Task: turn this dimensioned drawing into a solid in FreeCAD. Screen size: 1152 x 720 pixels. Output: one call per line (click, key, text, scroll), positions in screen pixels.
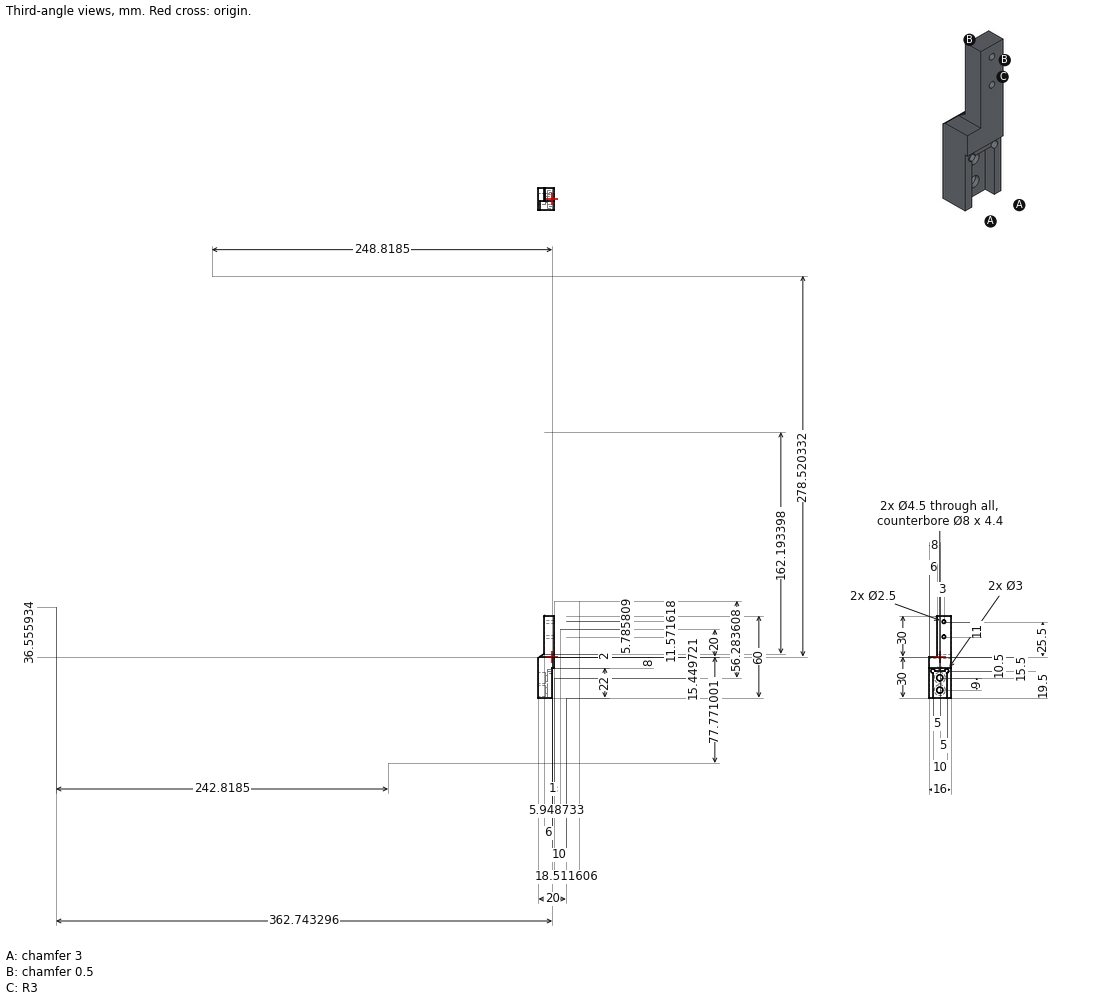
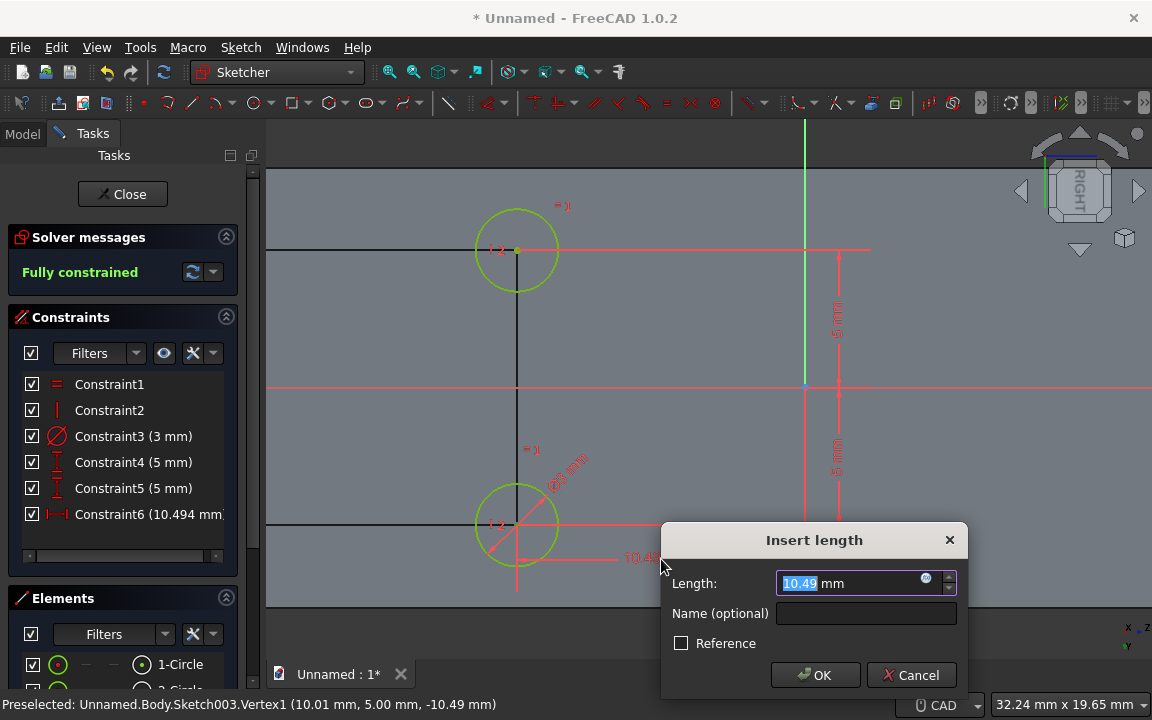
text(10.5)
key(Return)
key(Escape)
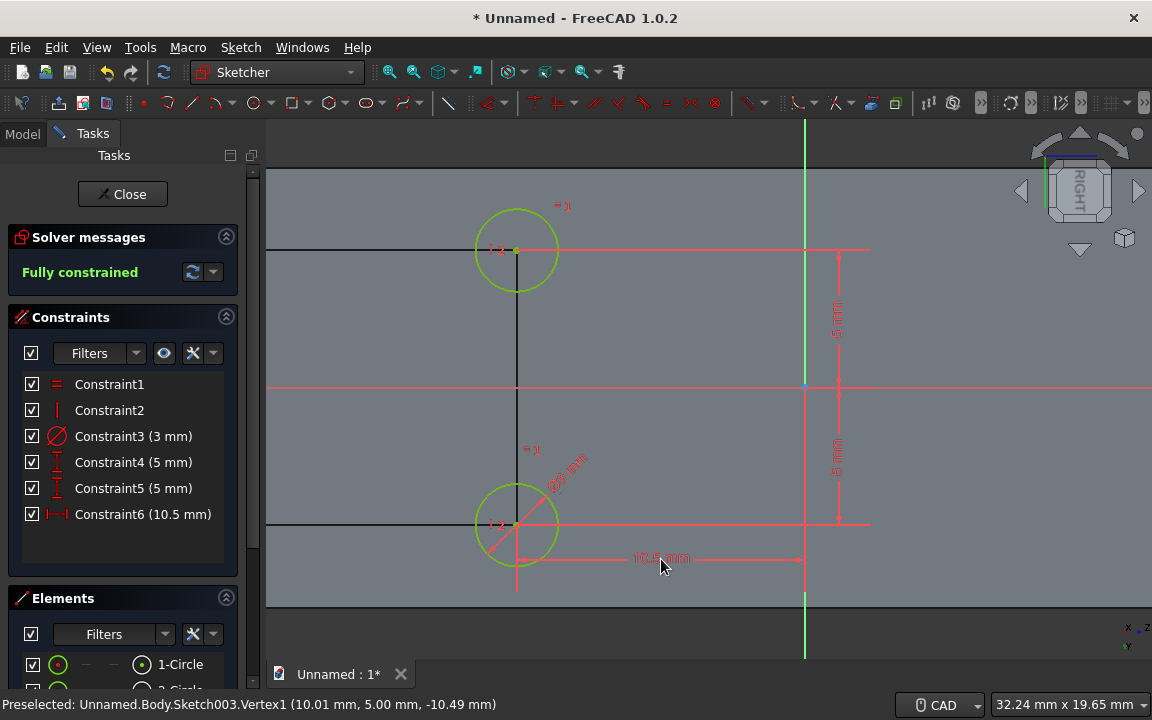
click(123, 194)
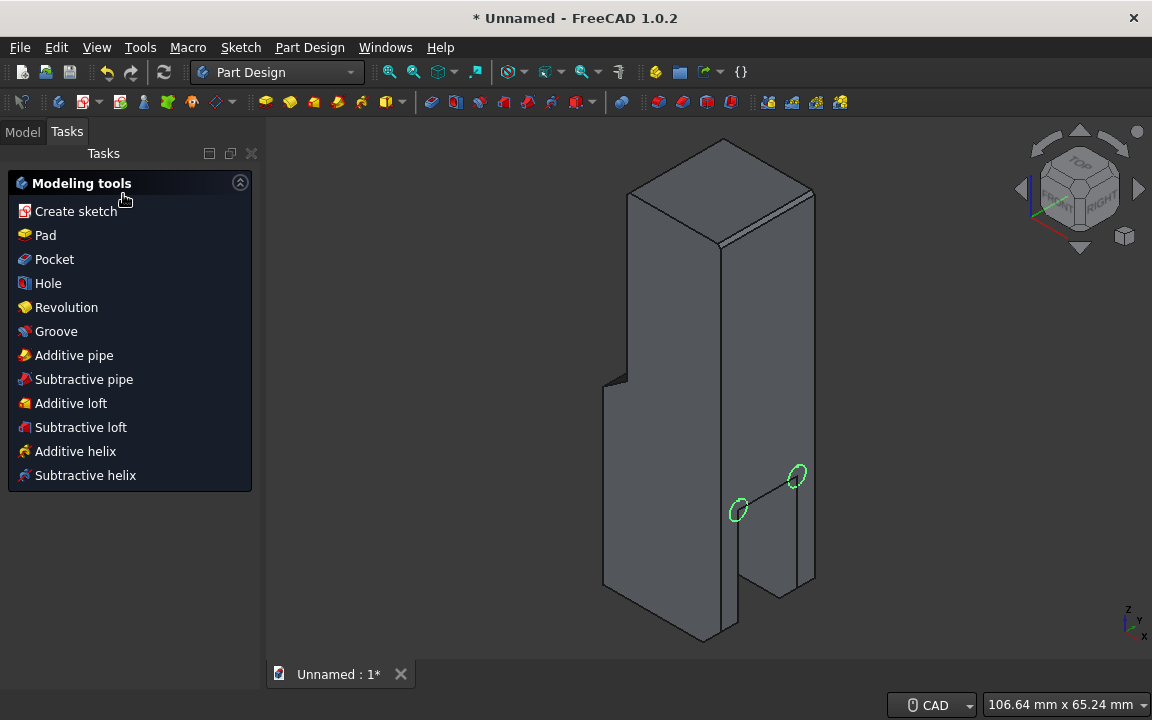
click(432, 102)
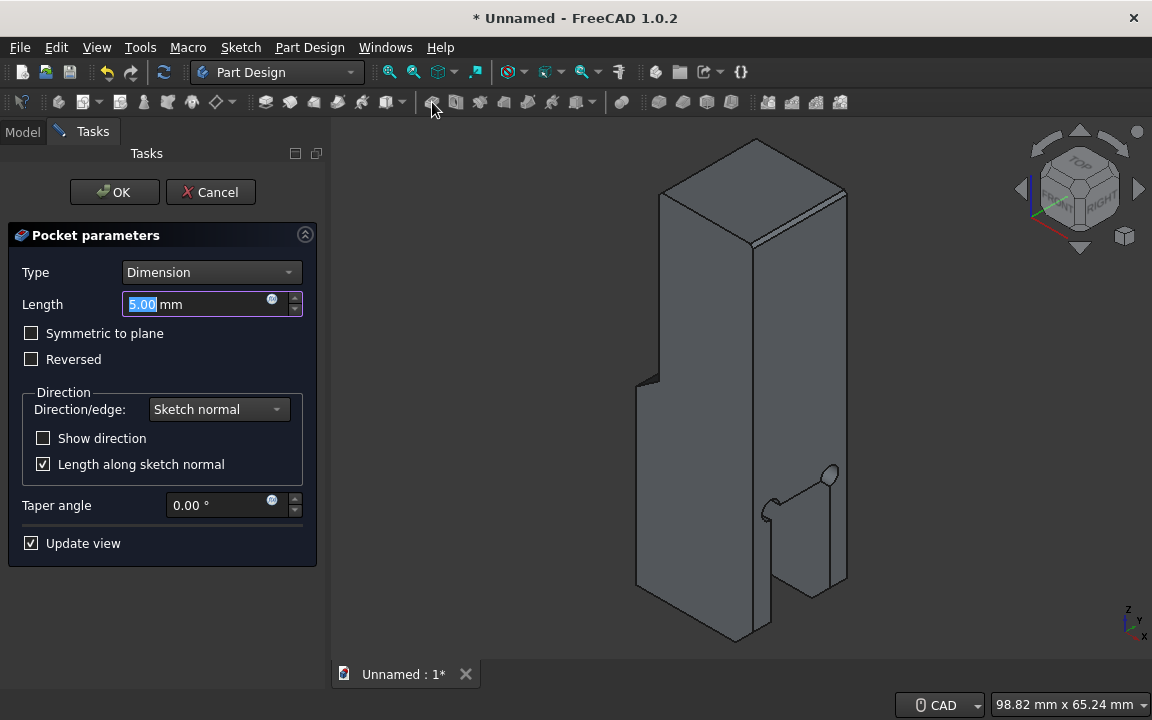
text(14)
key(Tab)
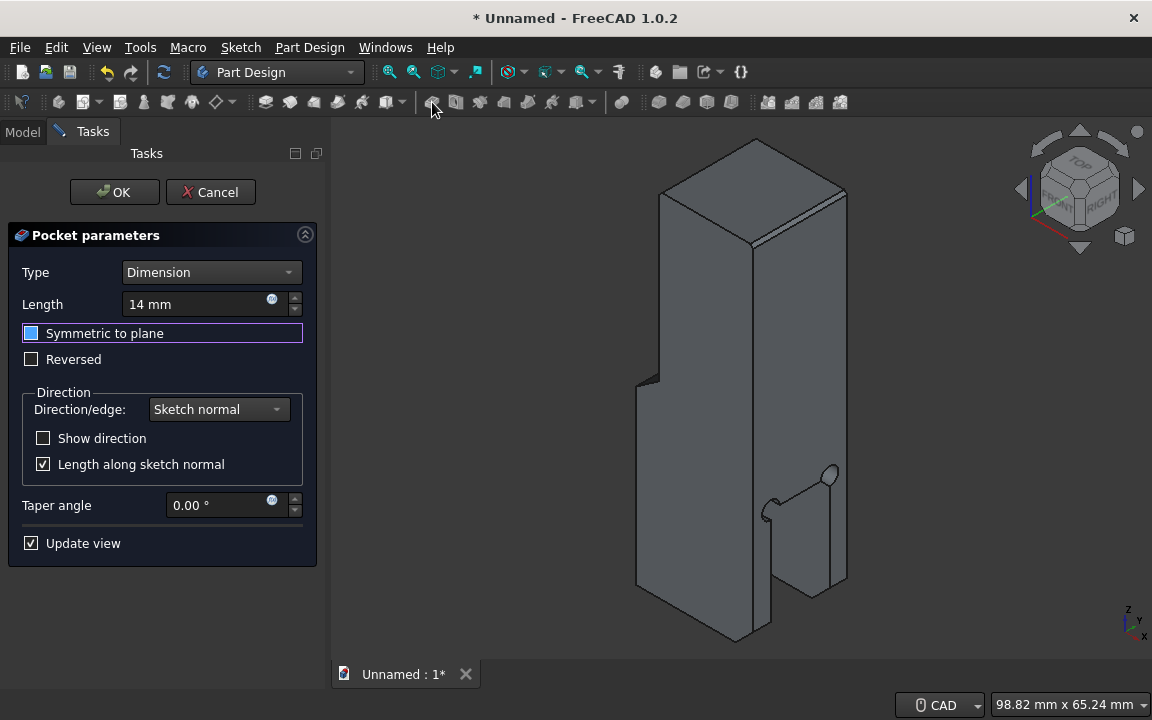
click(115, 192)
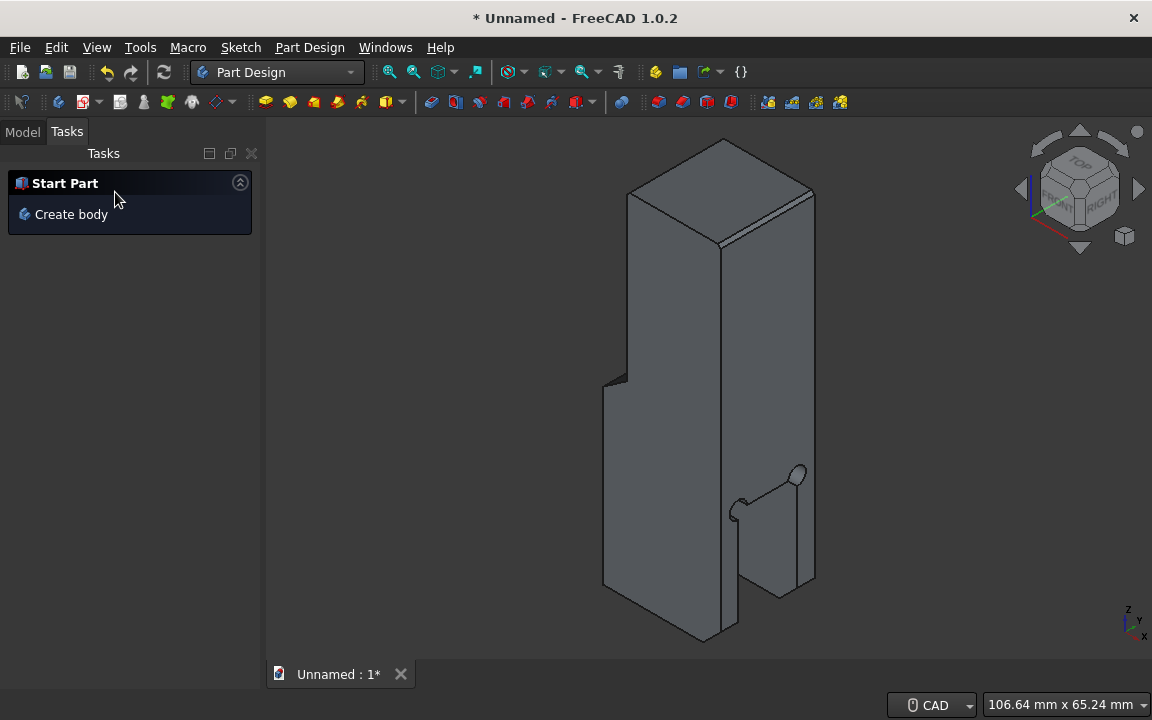
key(6)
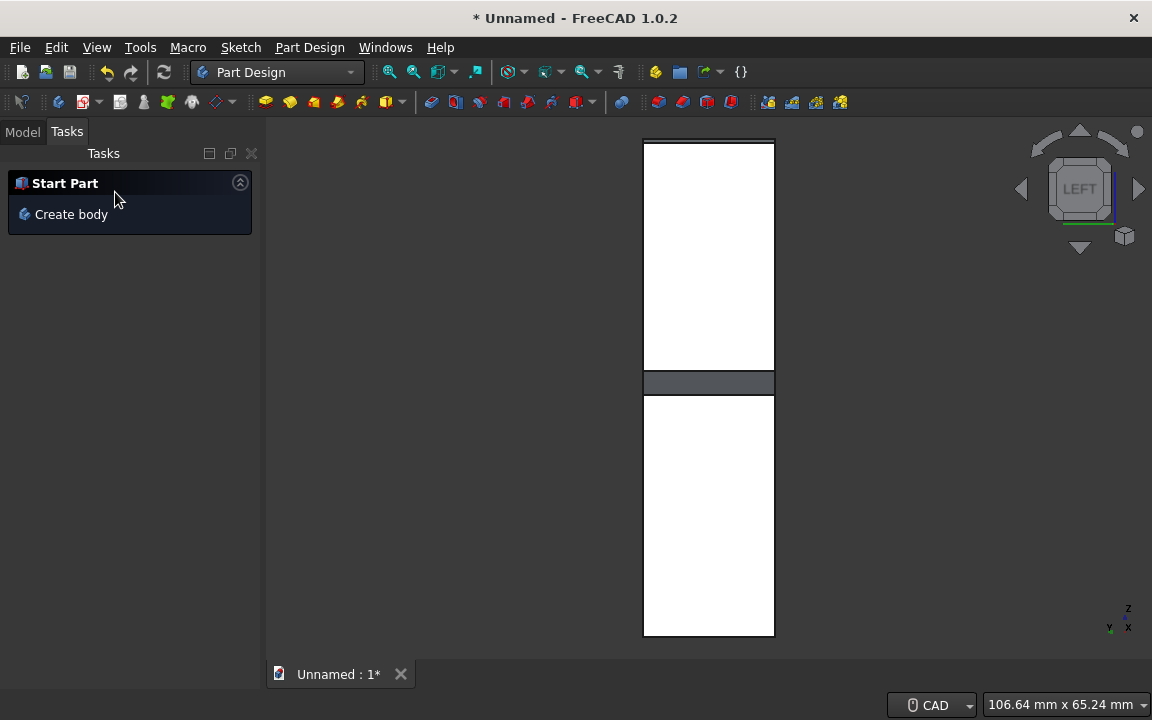
click(709, 480)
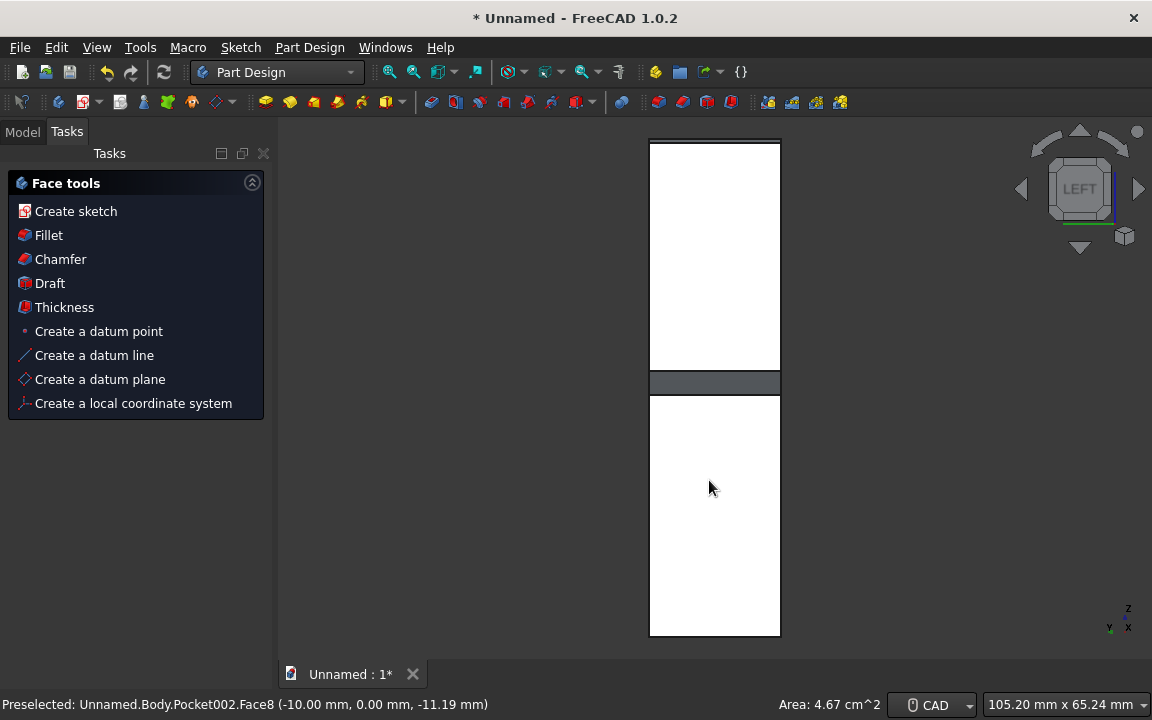
click(84, 102)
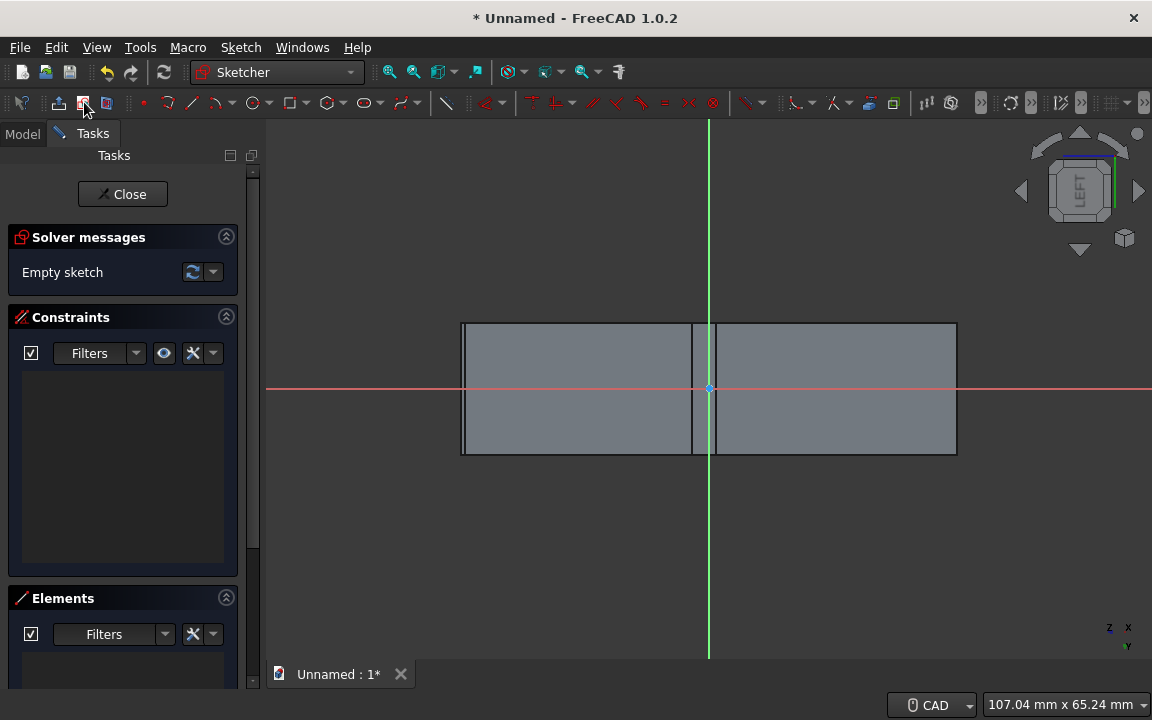
scroll(966, 389, up, 4)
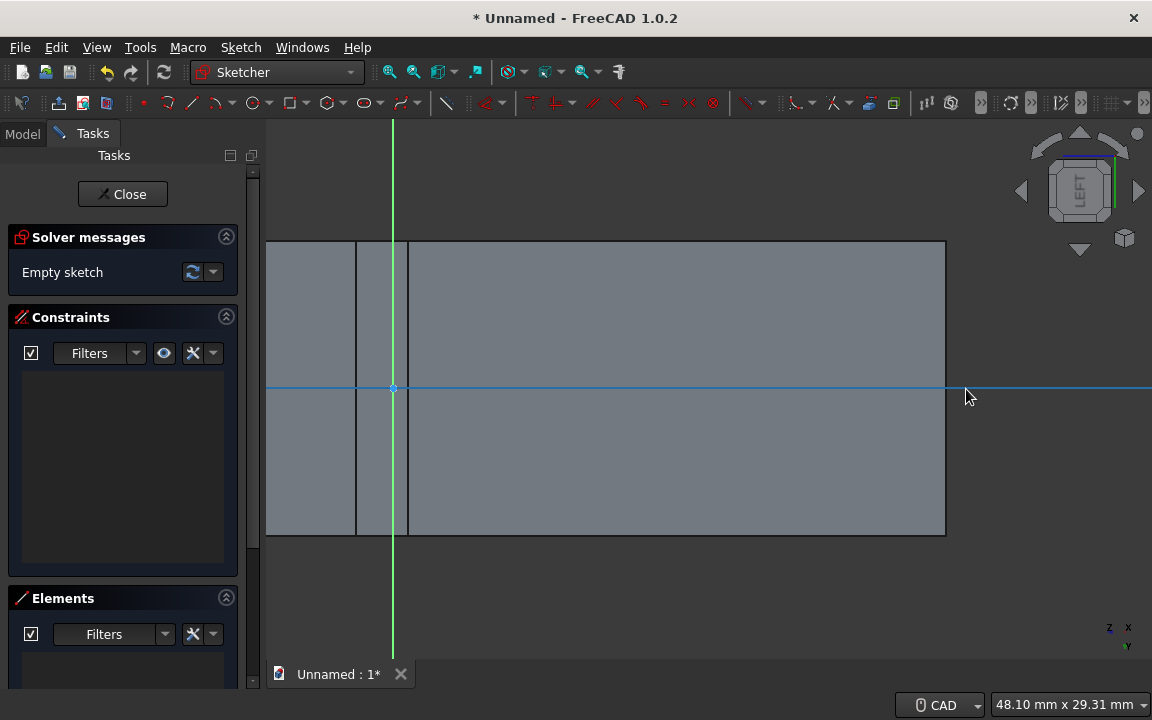
click(254, 104)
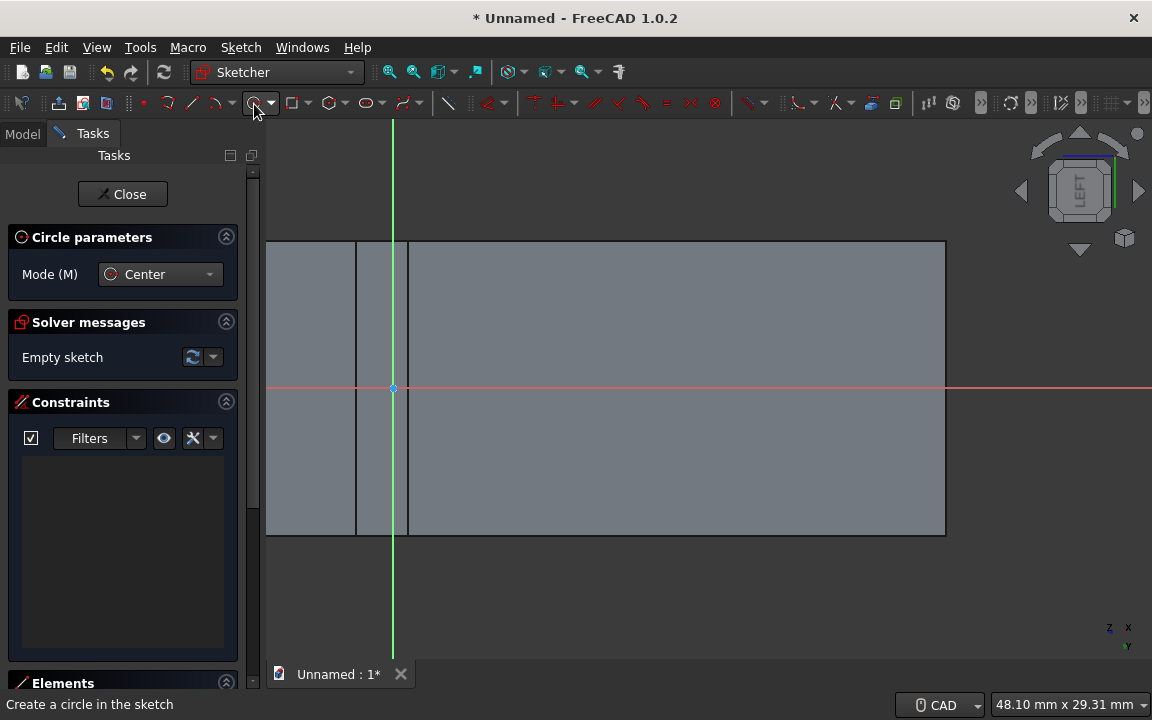
click(679, 388)
click(708, 359)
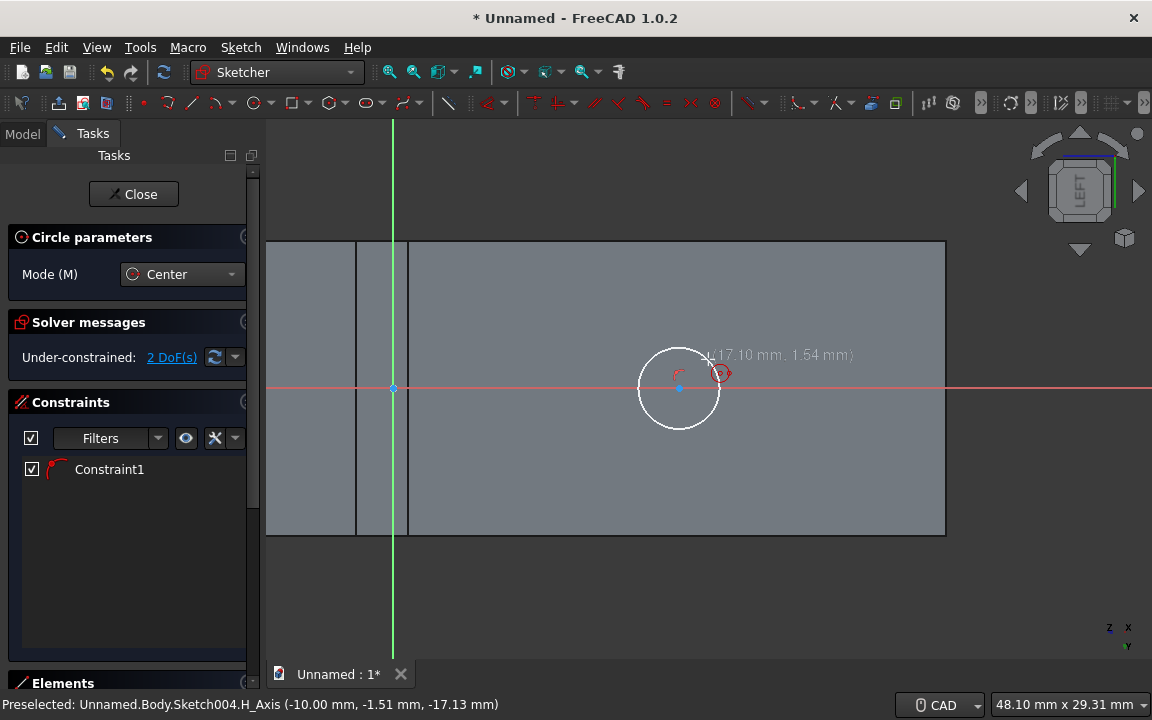
click(844, 388)
click(874, 359)
key(Escape)